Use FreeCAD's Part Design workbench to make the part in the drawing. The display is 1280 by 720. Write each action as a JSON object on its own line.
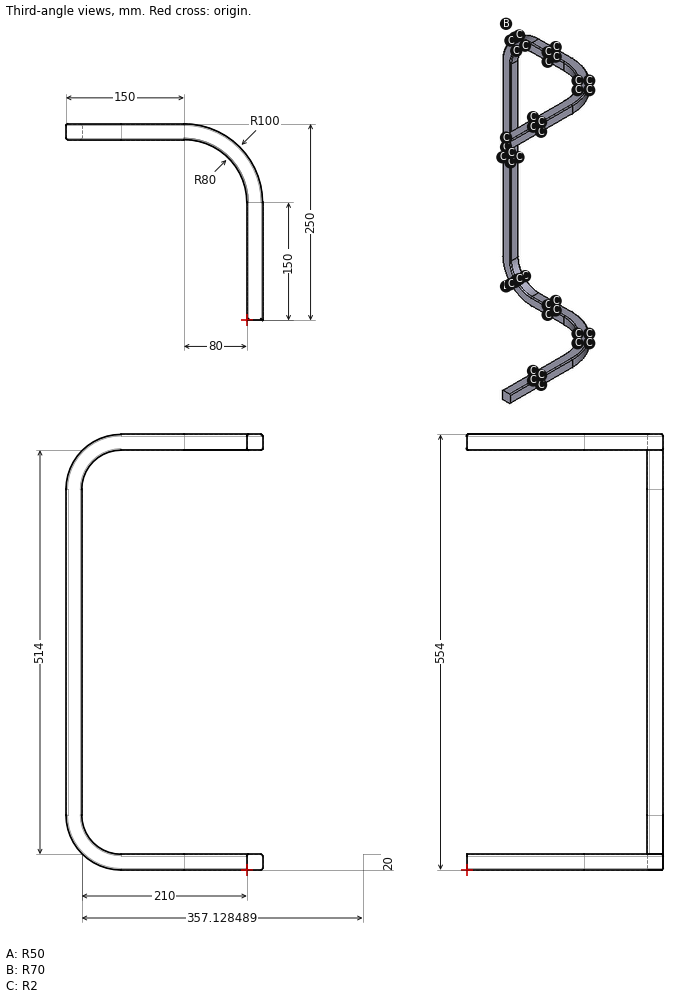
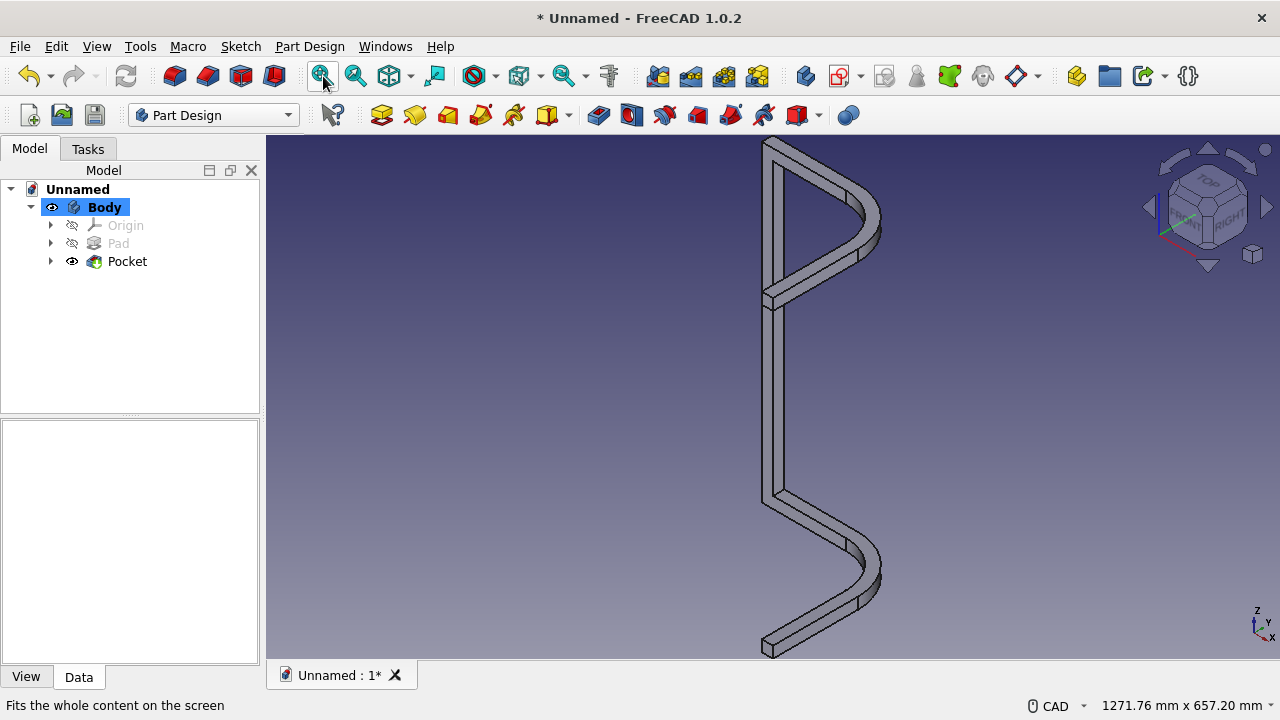
{"action": "left_click", "coordinate": [323, 76]}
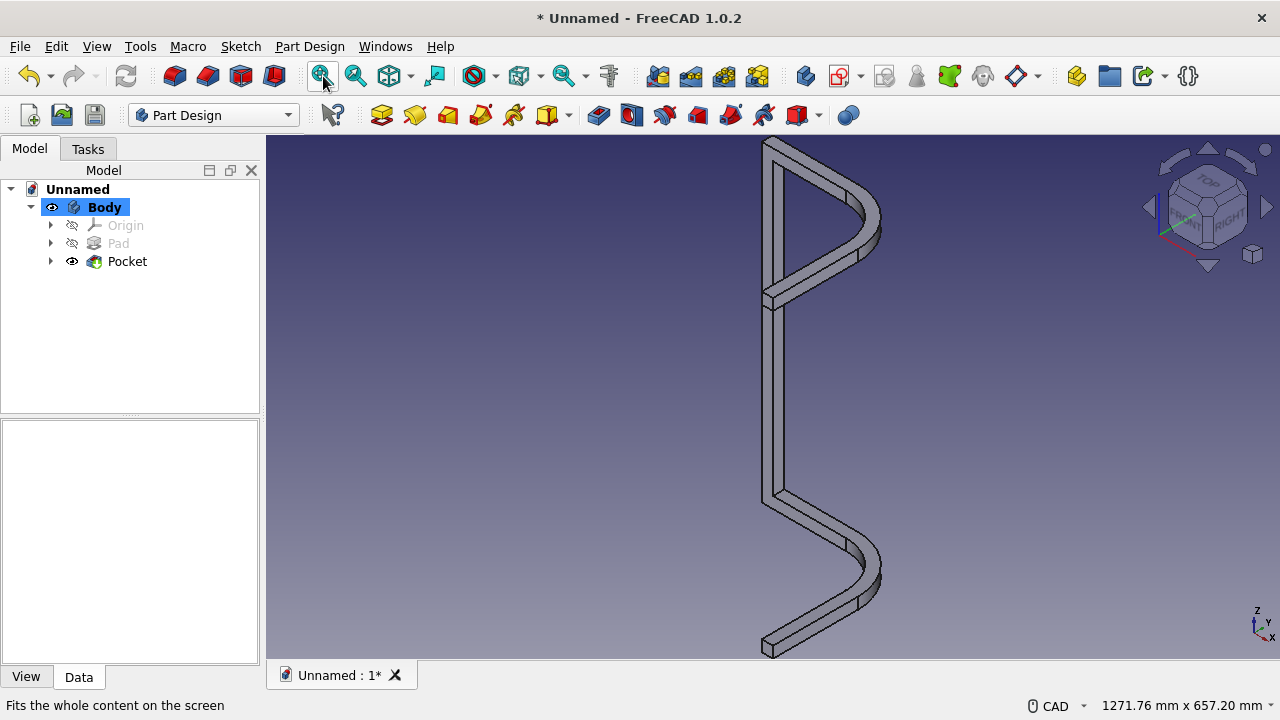
{"action": "key", "text": "2"}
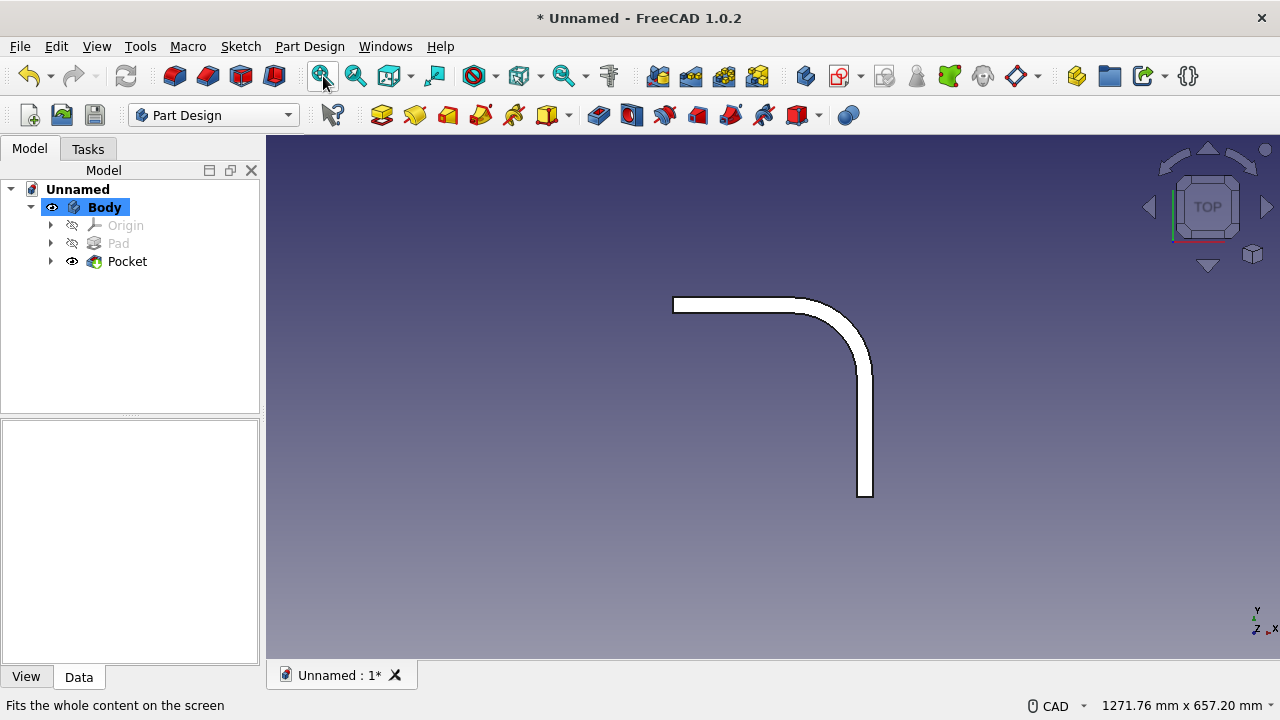
{"action": "left_click", "coordinate": [323, 76]}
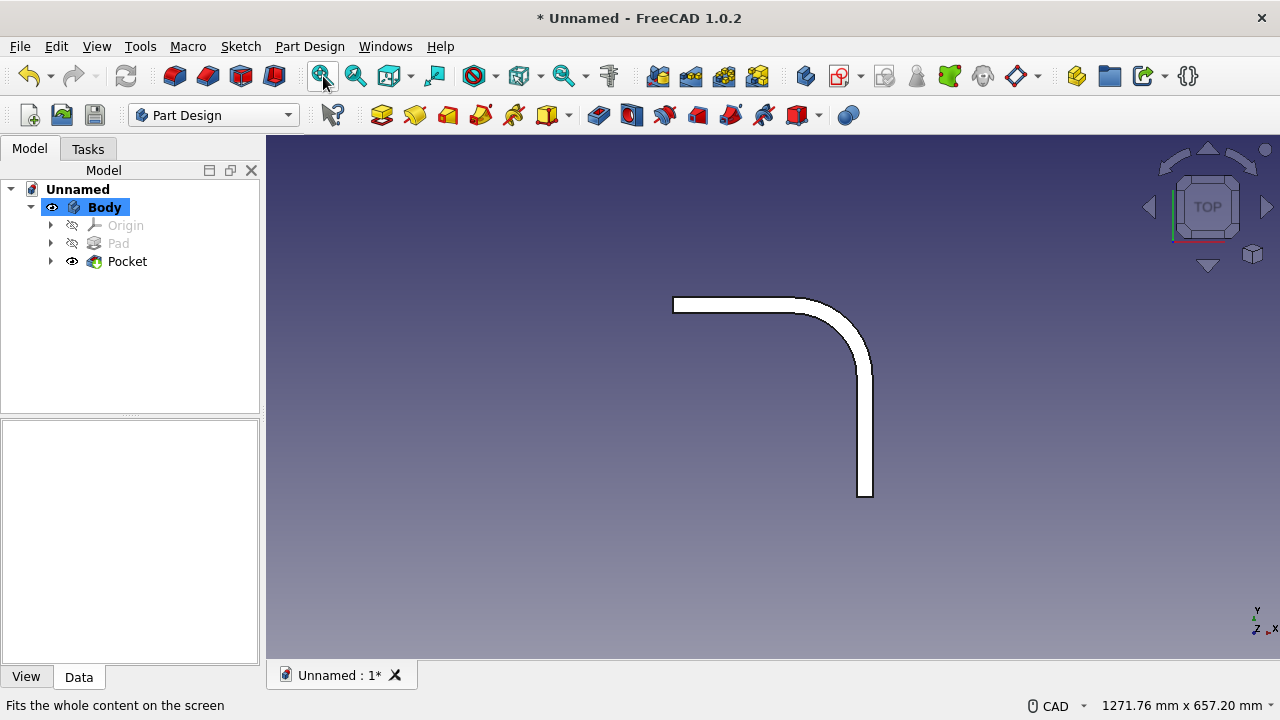
{"action": "scroll", "coordinate": [689, 304], "scroll_direction": "up", "scroll_amount": 5}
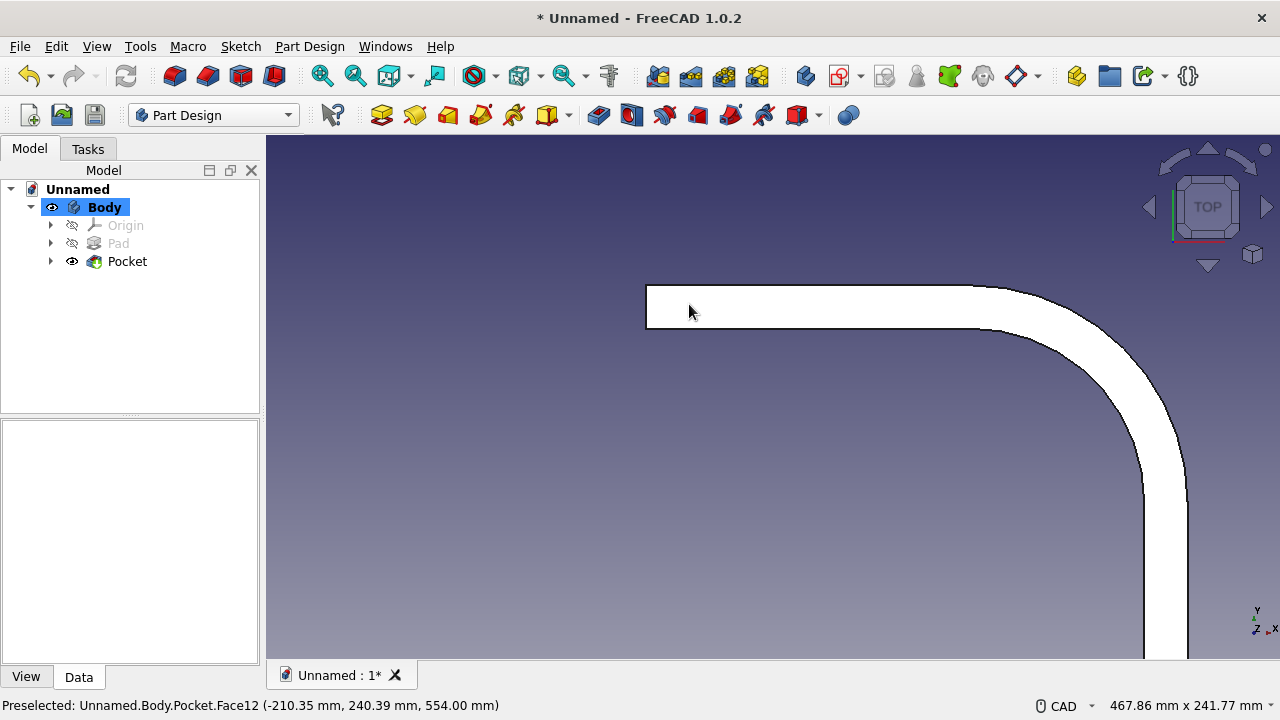
{"action": "left_click", "coordinate": [323, 76]}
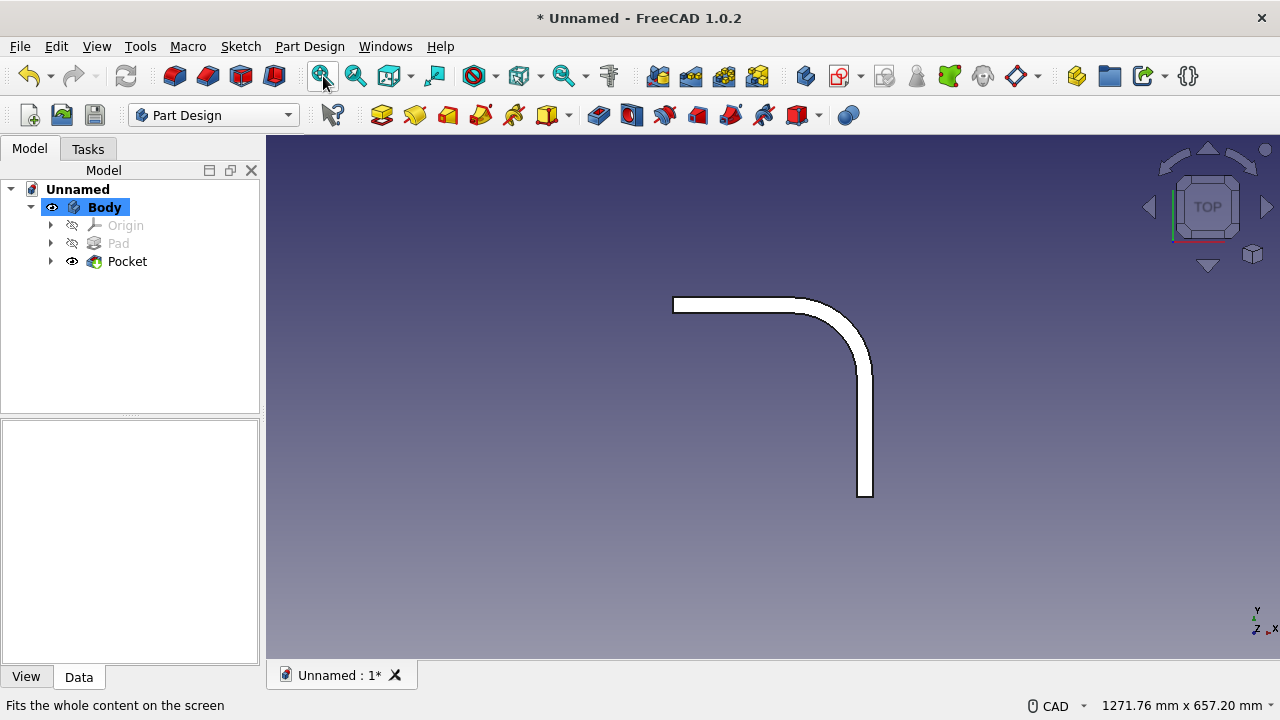
{"action": "key", "text": "1"}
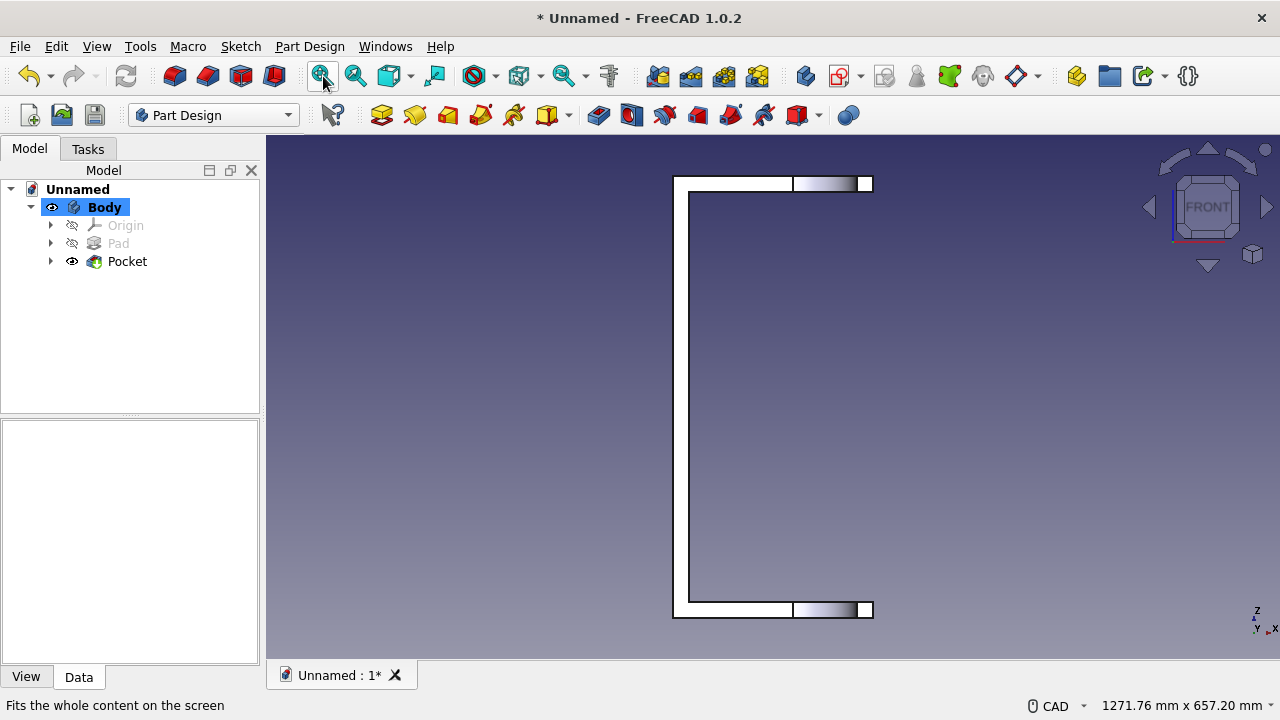
{"action": "scroll", "coordinate": [689, 191], "scroll_direction": "up", "scroll_amount": 5}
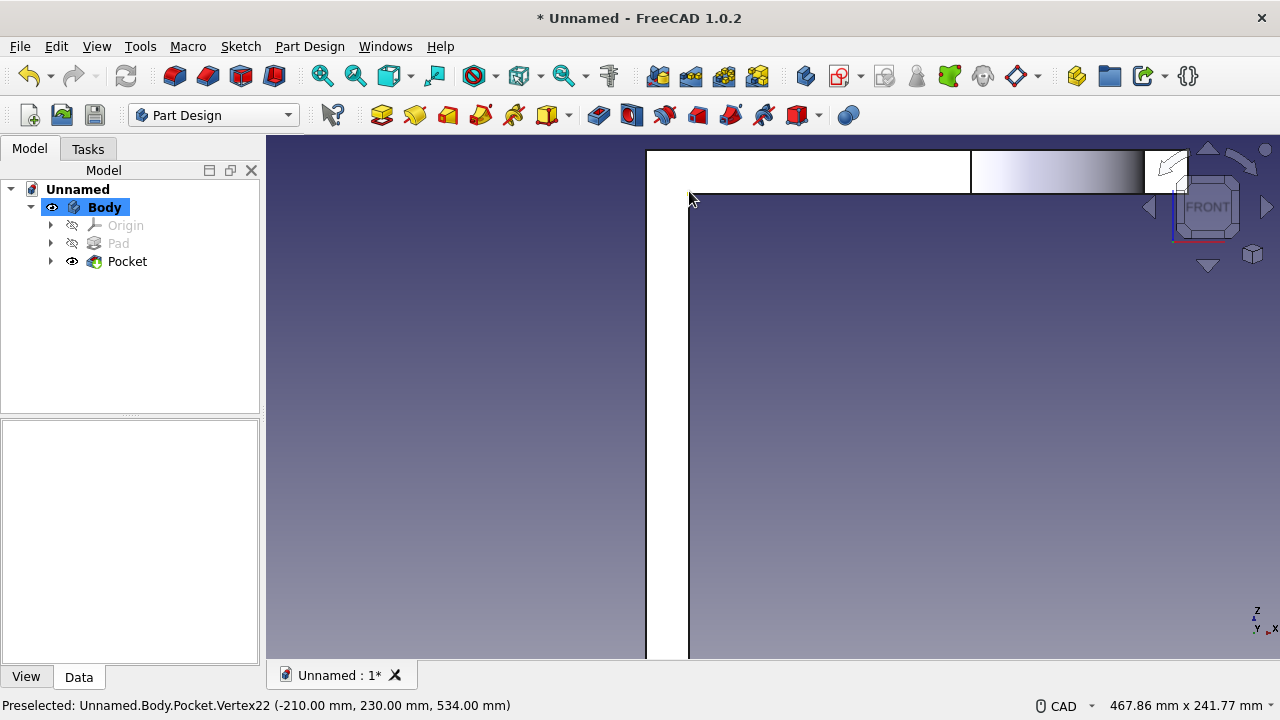
{"action": "left_click", "coordinate": [323, 76]}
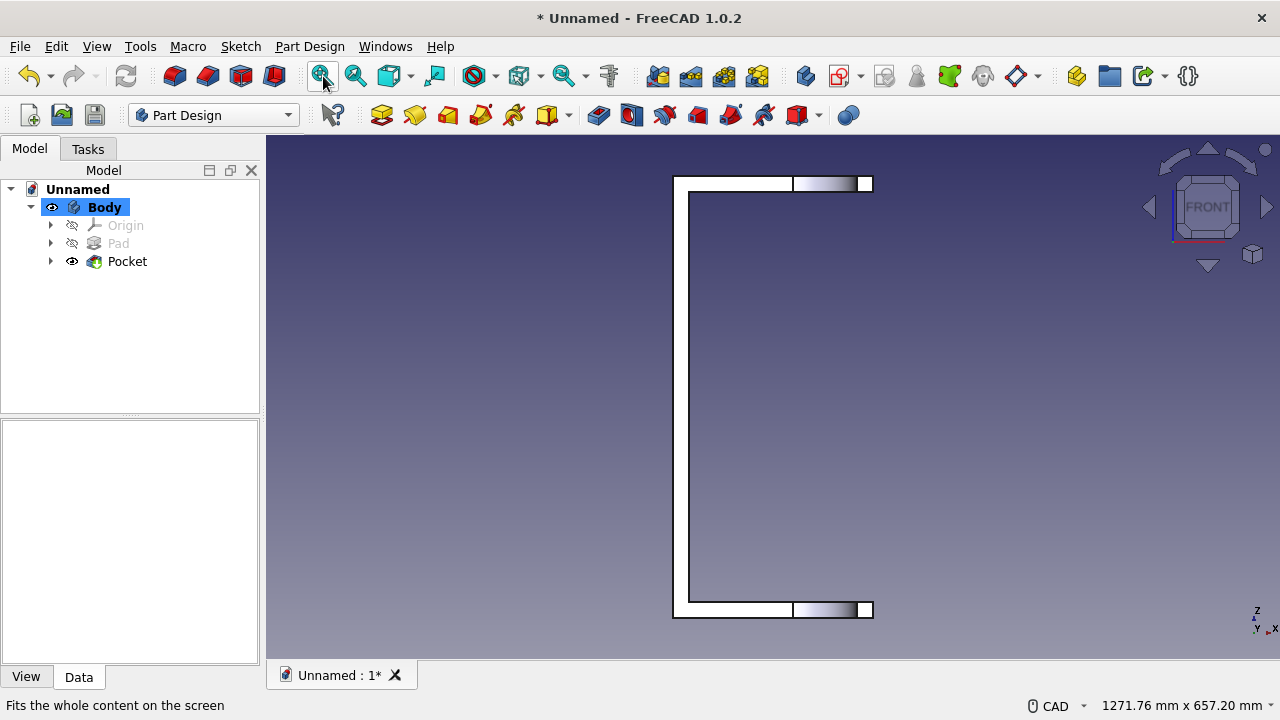
{"action": "key", "text": "3"}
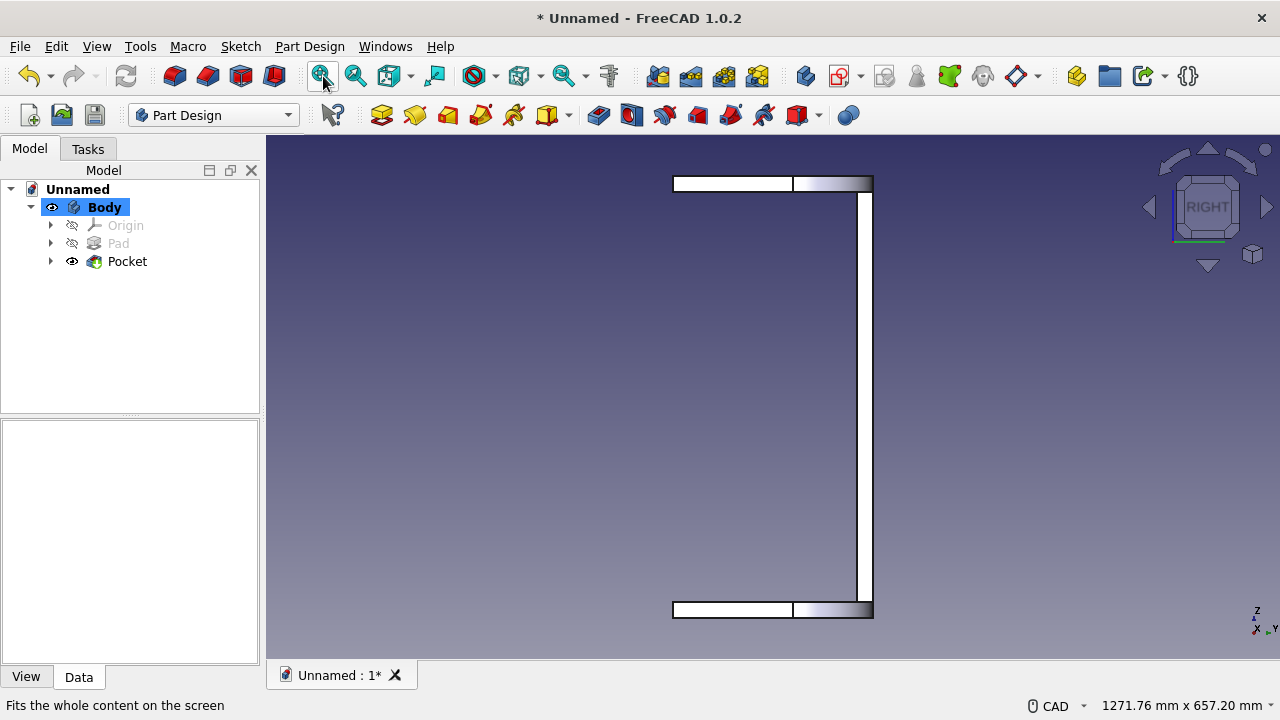
{"action": "scroll", "coordinate": [865, 191], "scroll_direction": "up", "scroll_amount": 5}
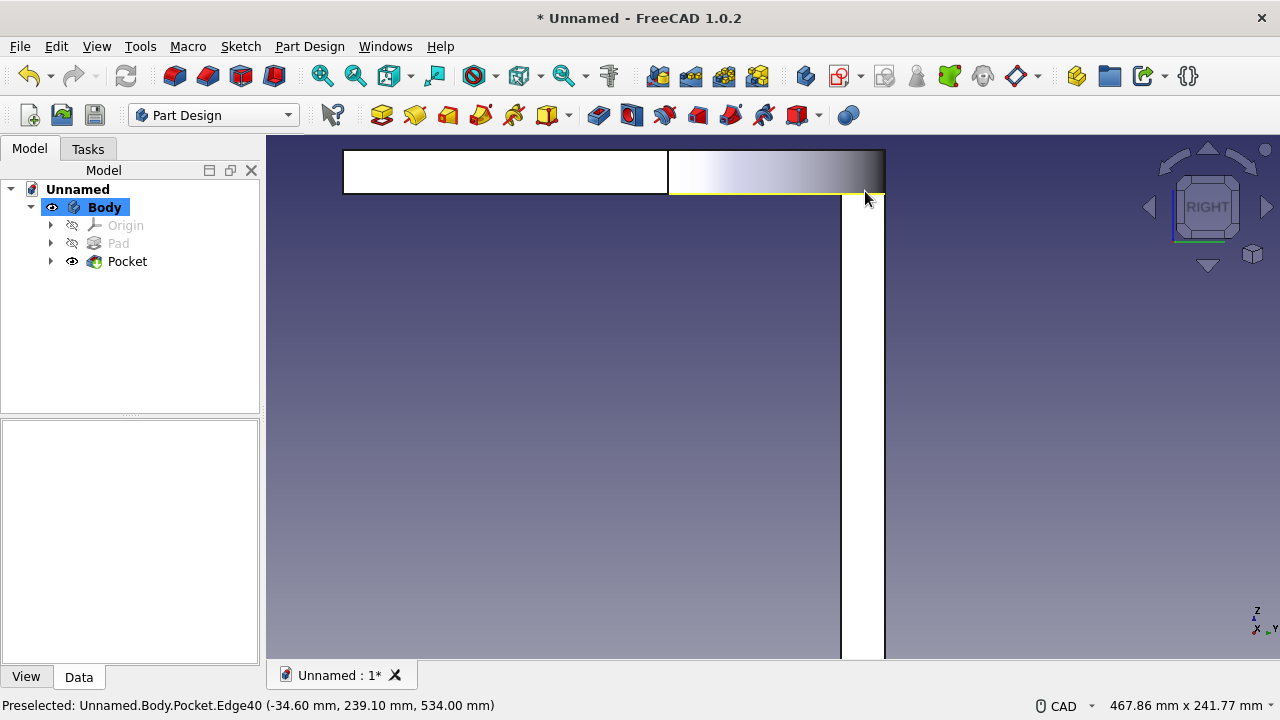
{"action": "left_click", "coordinate": [323, 76]}